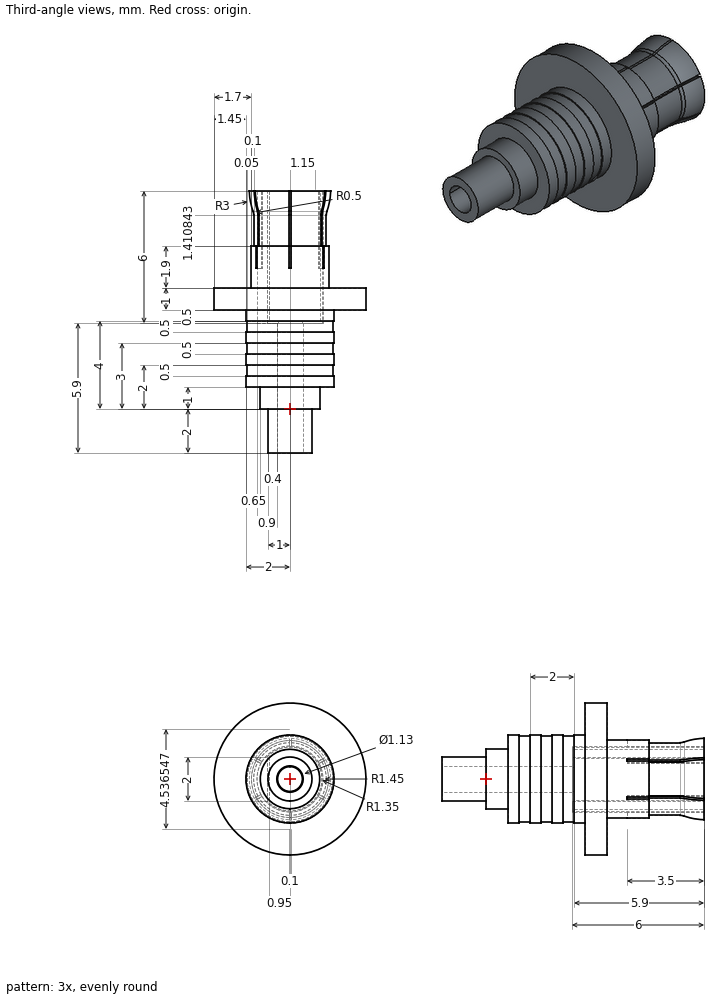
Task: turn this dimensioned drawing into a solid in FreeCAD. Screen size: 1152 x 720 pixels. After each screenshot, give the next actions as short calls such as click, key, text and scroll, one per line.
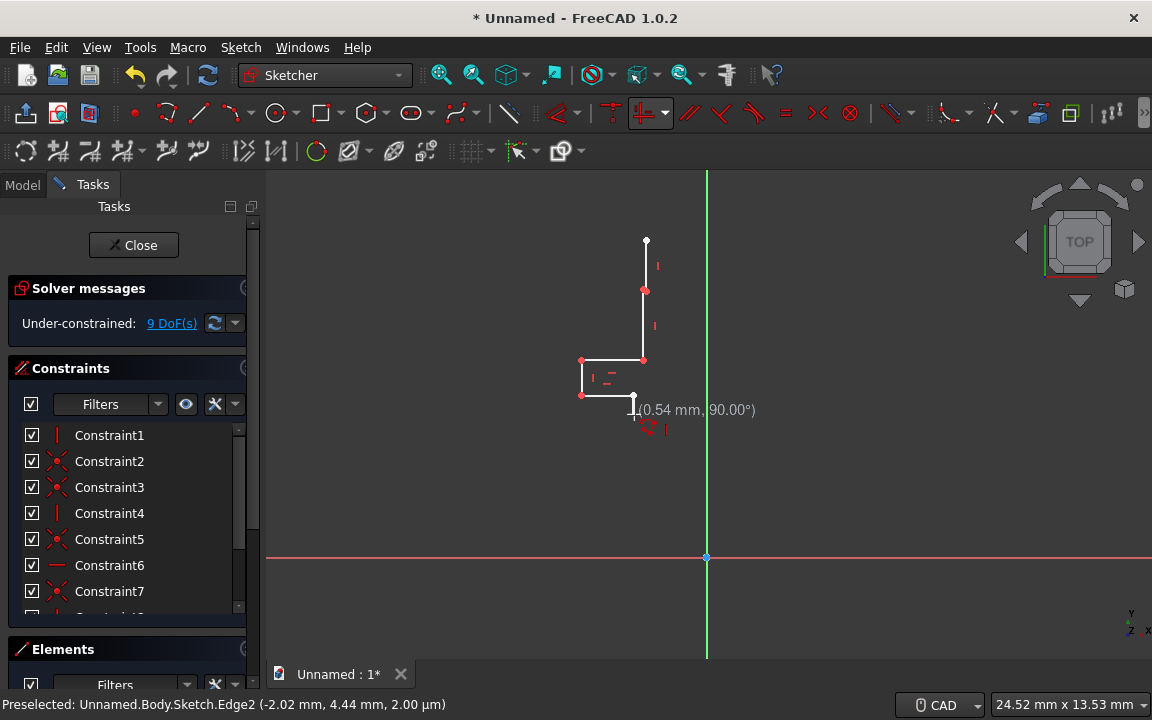
click(634, 413)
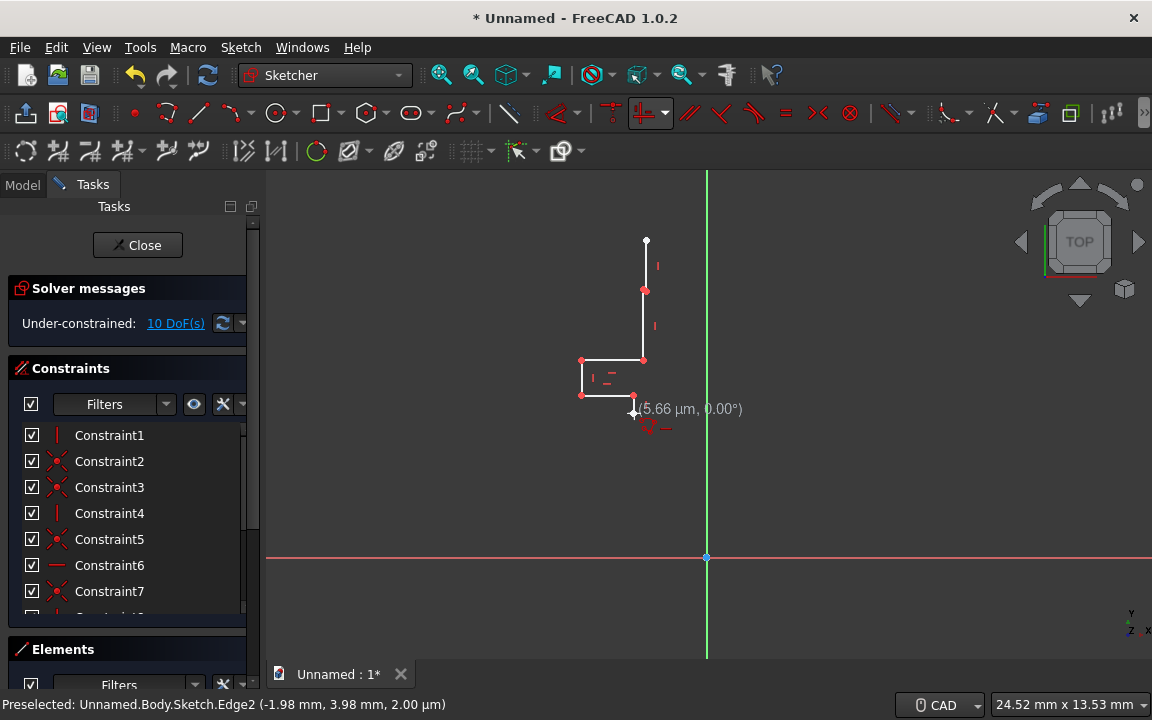
scroll(636, 413, up, 11)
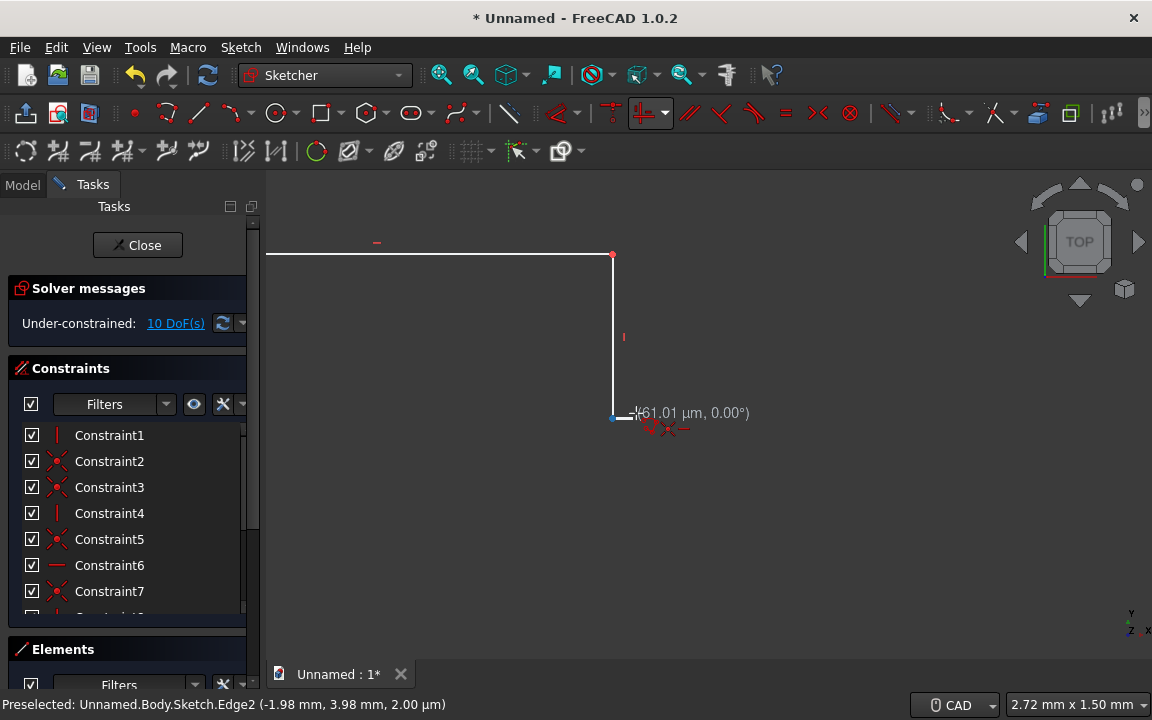
click(634, 409)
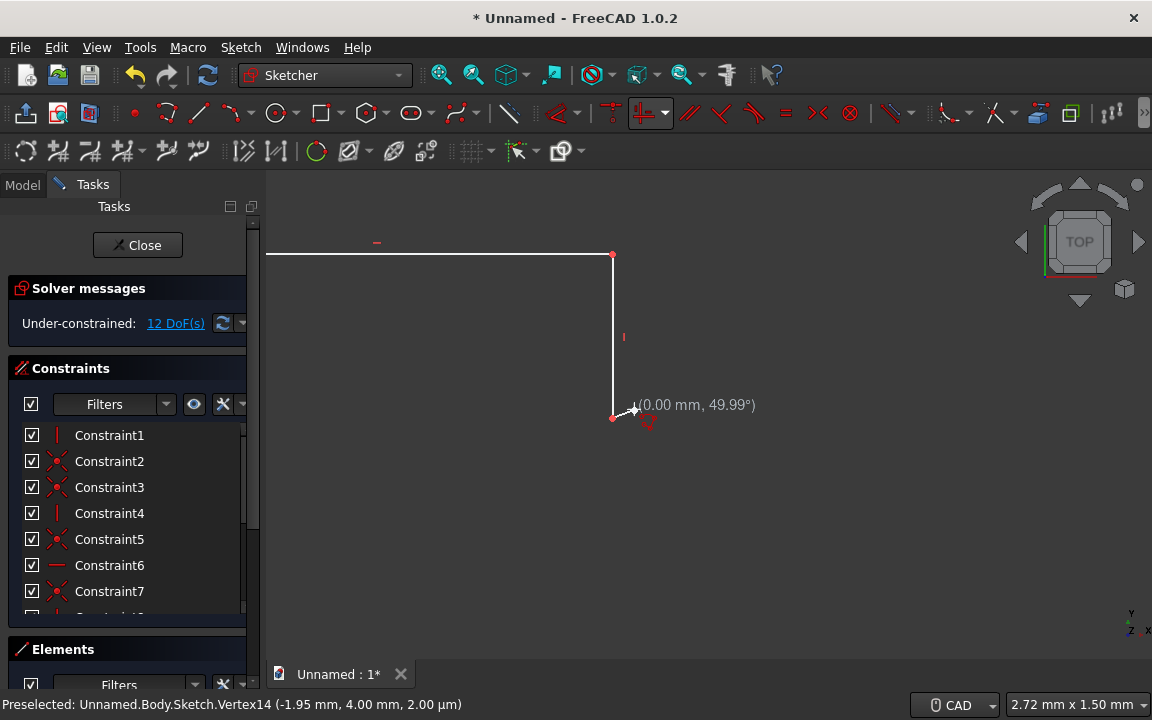
scroll(635, 414, down, 13)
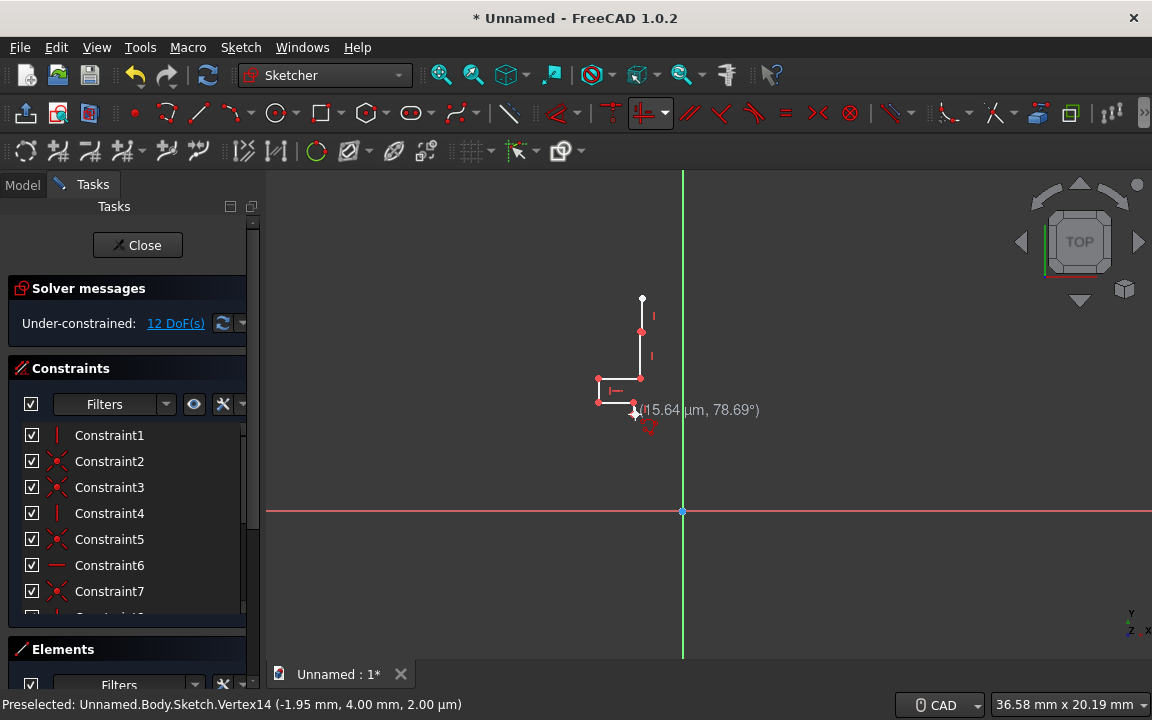
scroll(635, 426, up, 2)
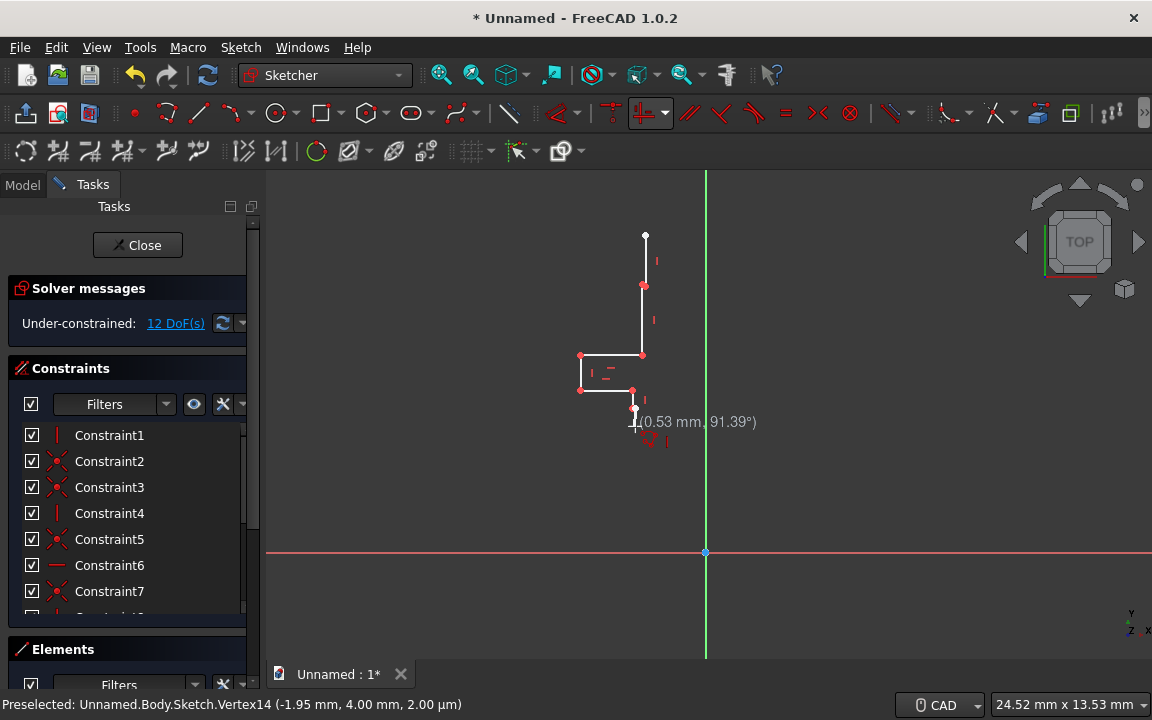
click(635, 426)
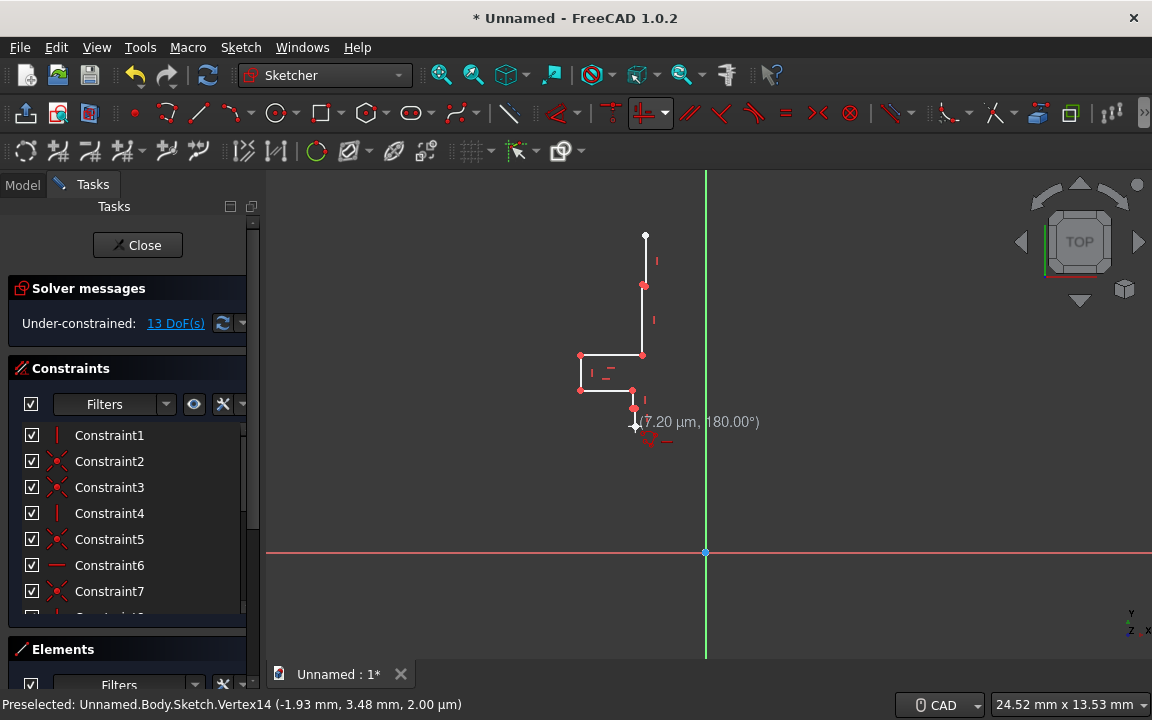
scroll(633, 426, up, 11)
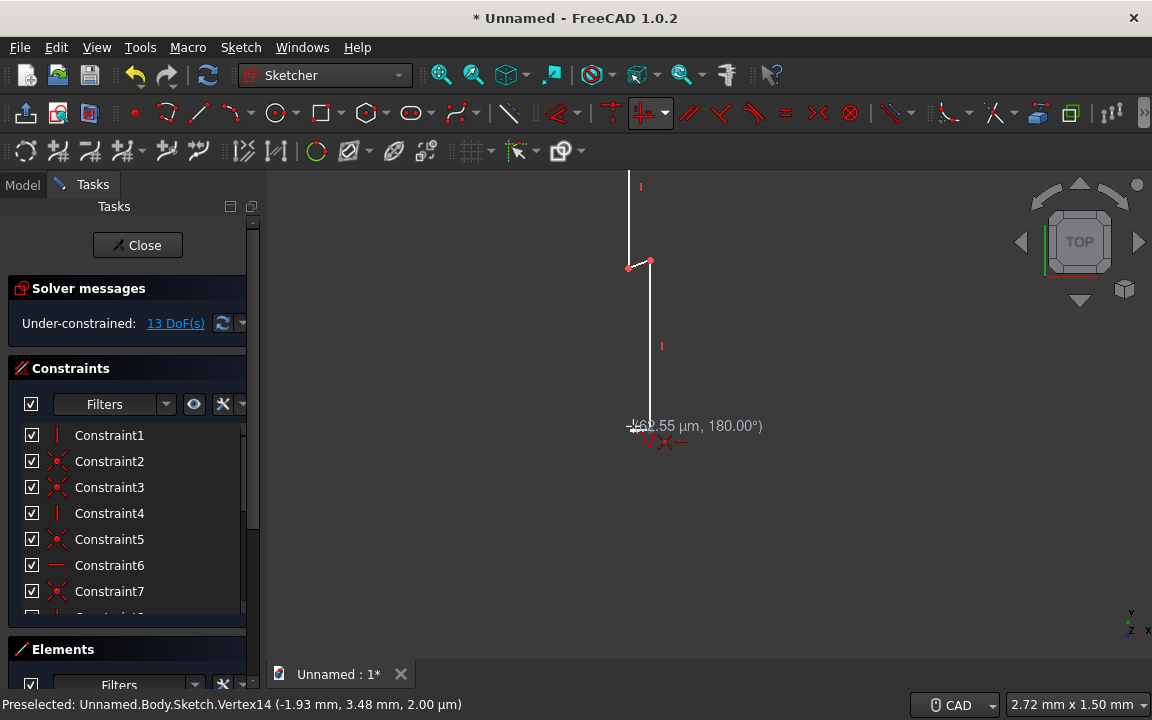
click(633, 422)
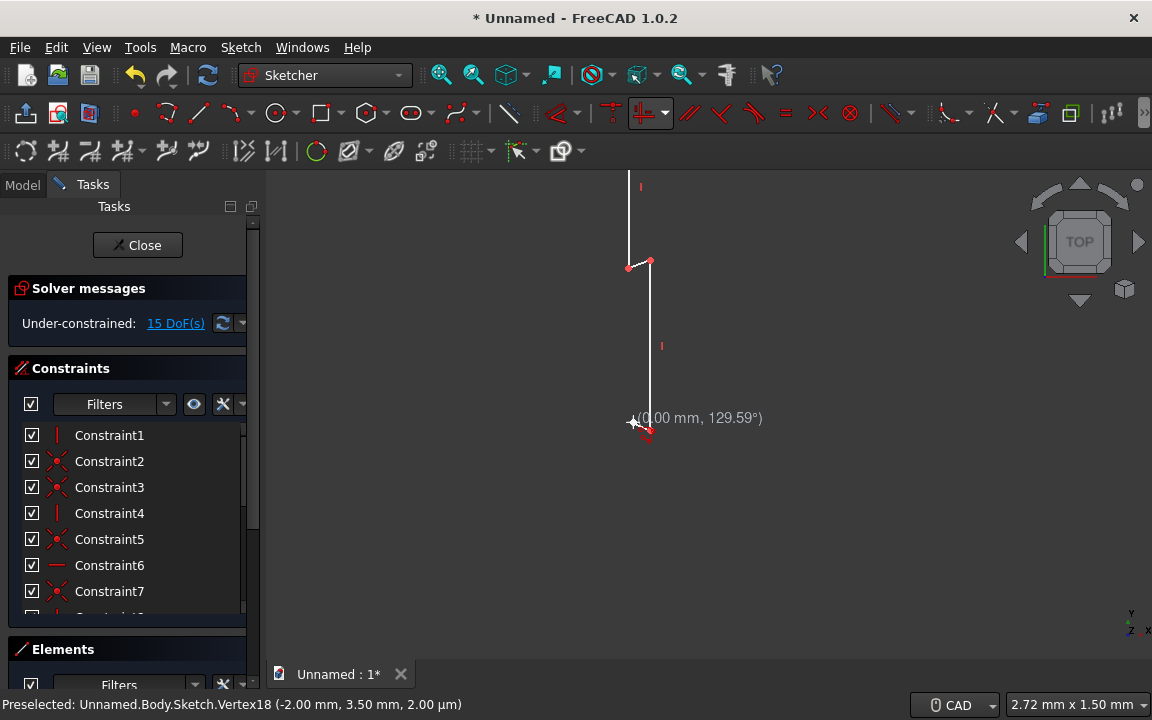
scroll(634, 426, down, 13)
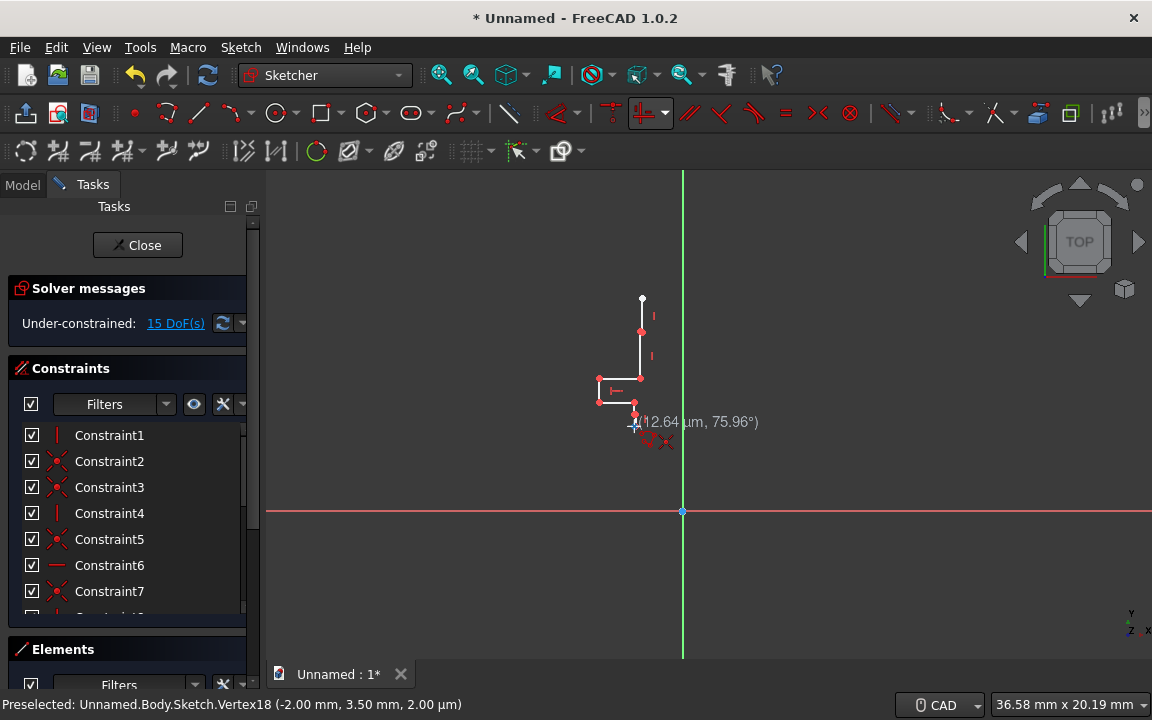
scroll(634, 438, up, 2)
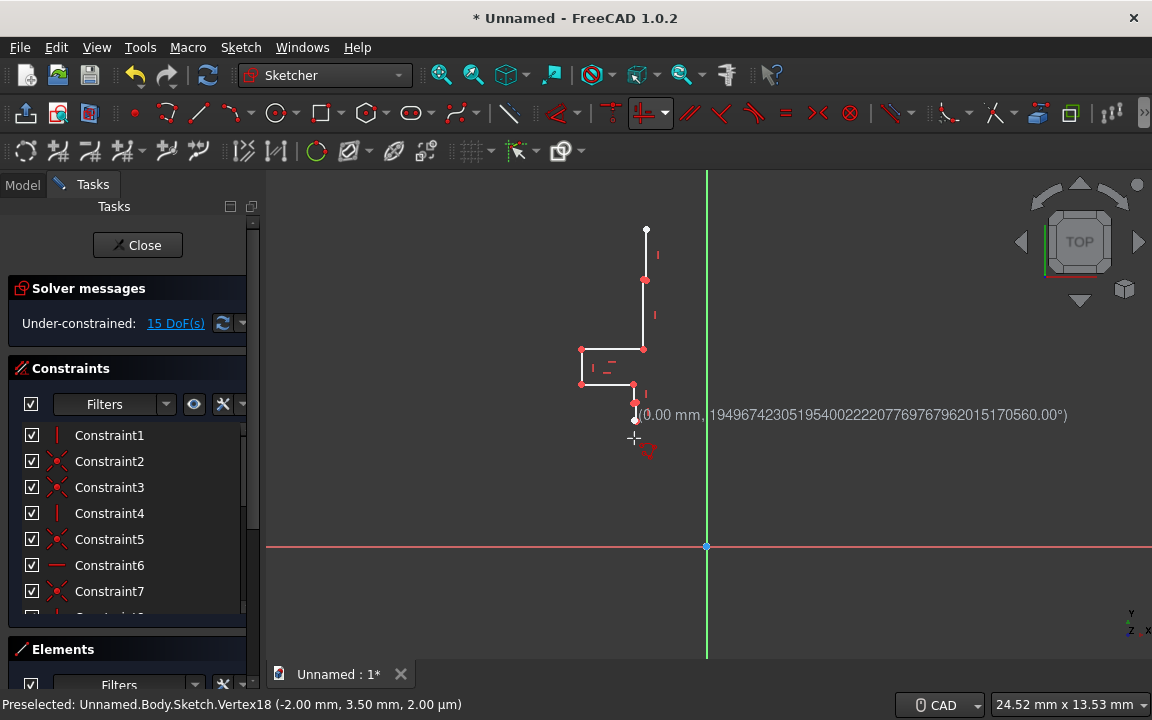
click(634, 438)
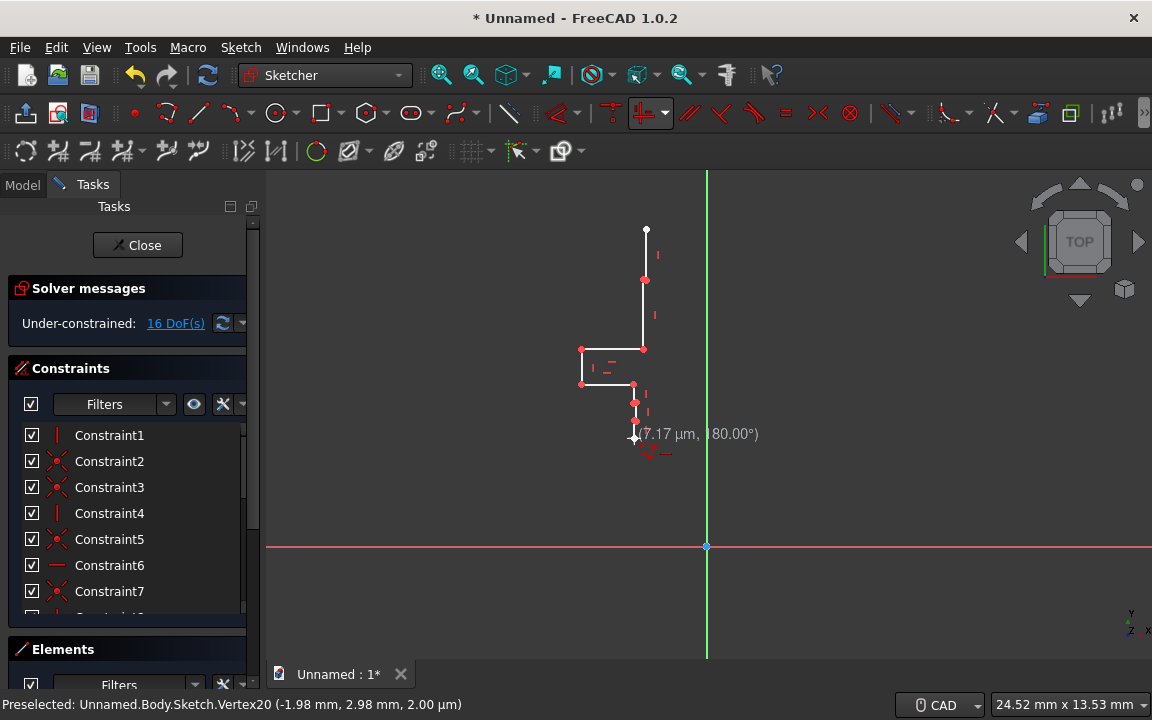
scroll(636, 438, up, 11)